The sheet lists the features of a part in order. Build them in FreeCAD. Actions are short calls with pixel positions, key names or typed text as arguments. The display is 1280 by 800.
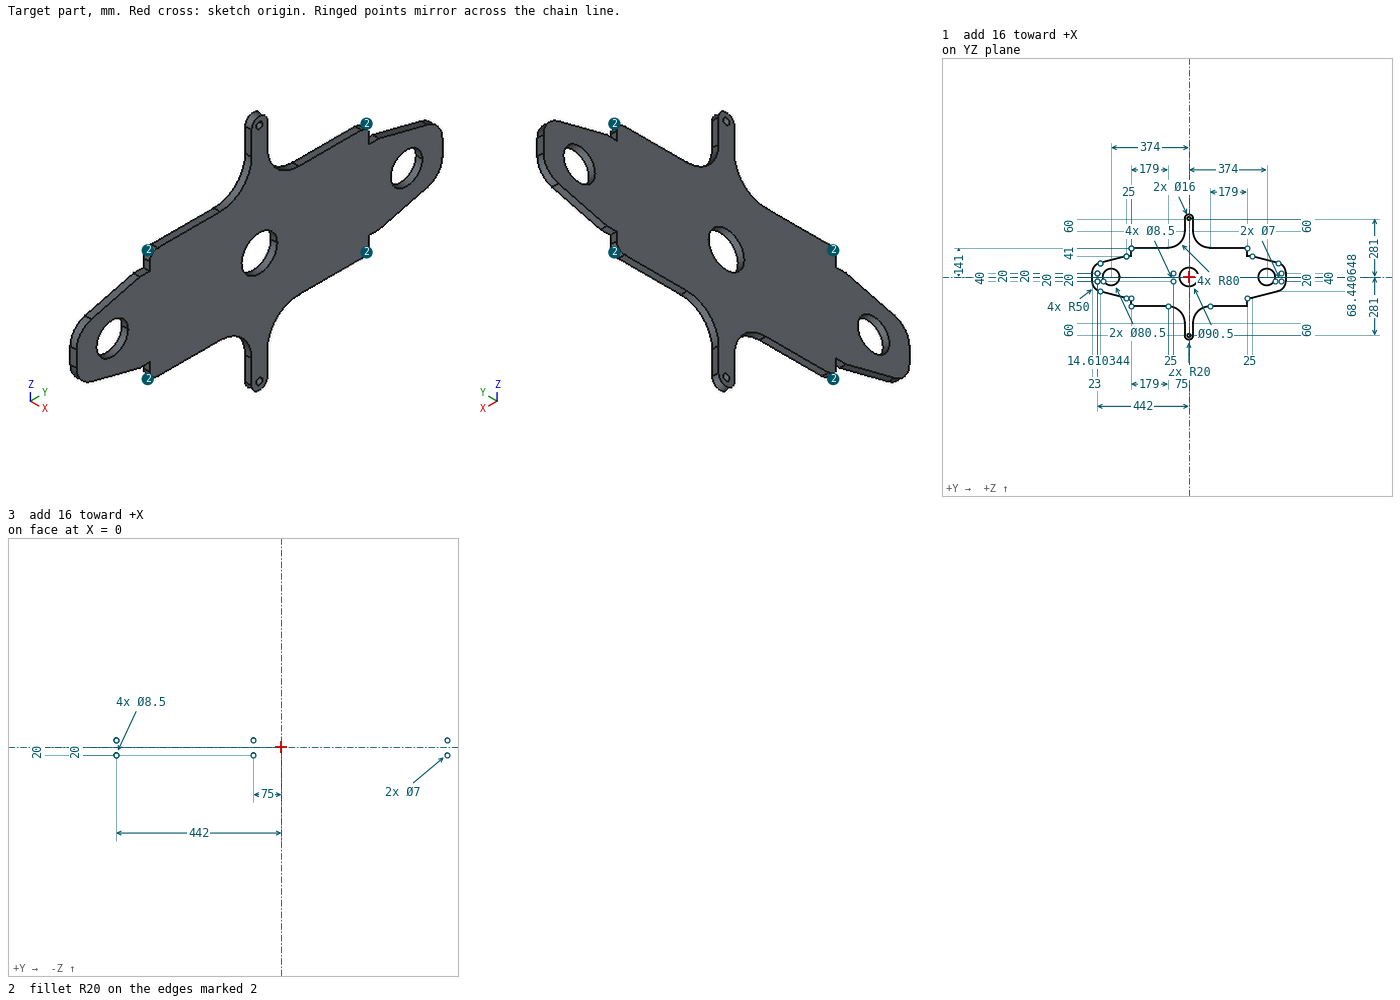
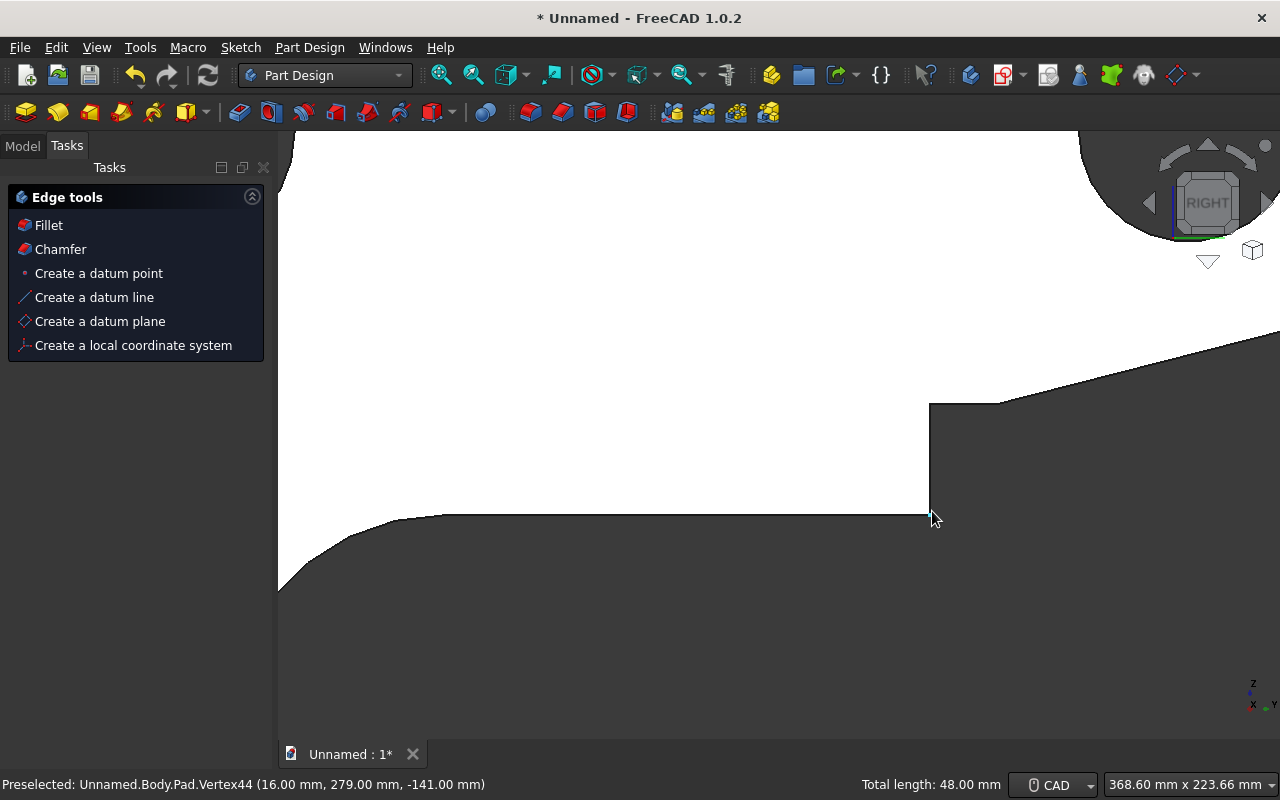
key(v)
key(f)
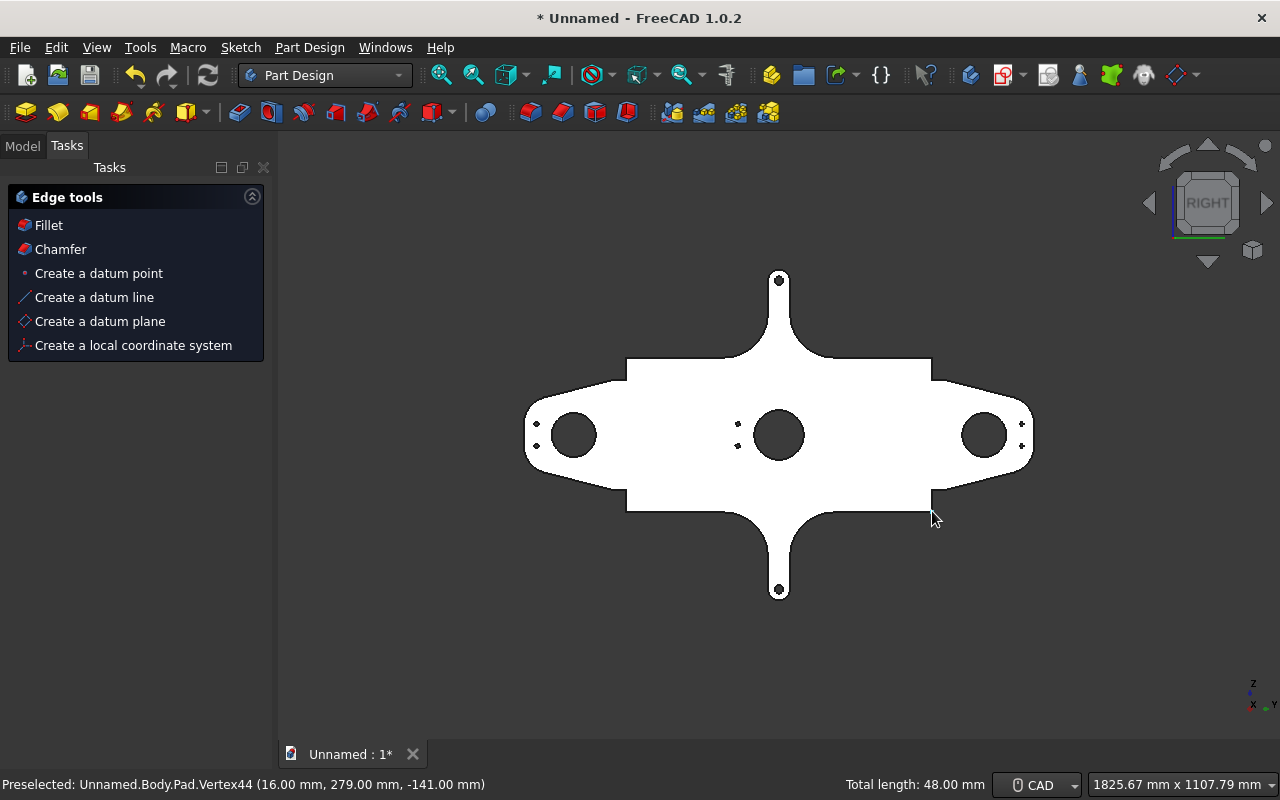
key(5)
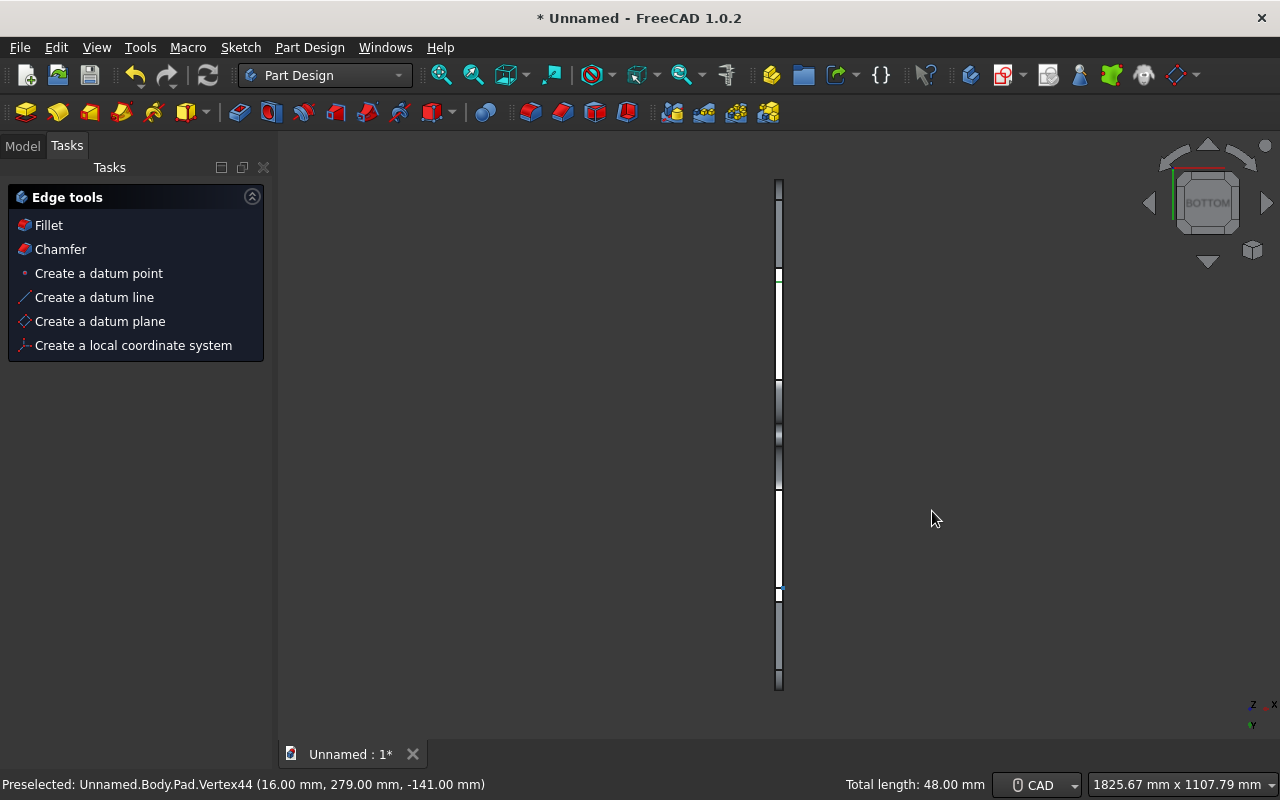
scroll(779, 587, up, 8)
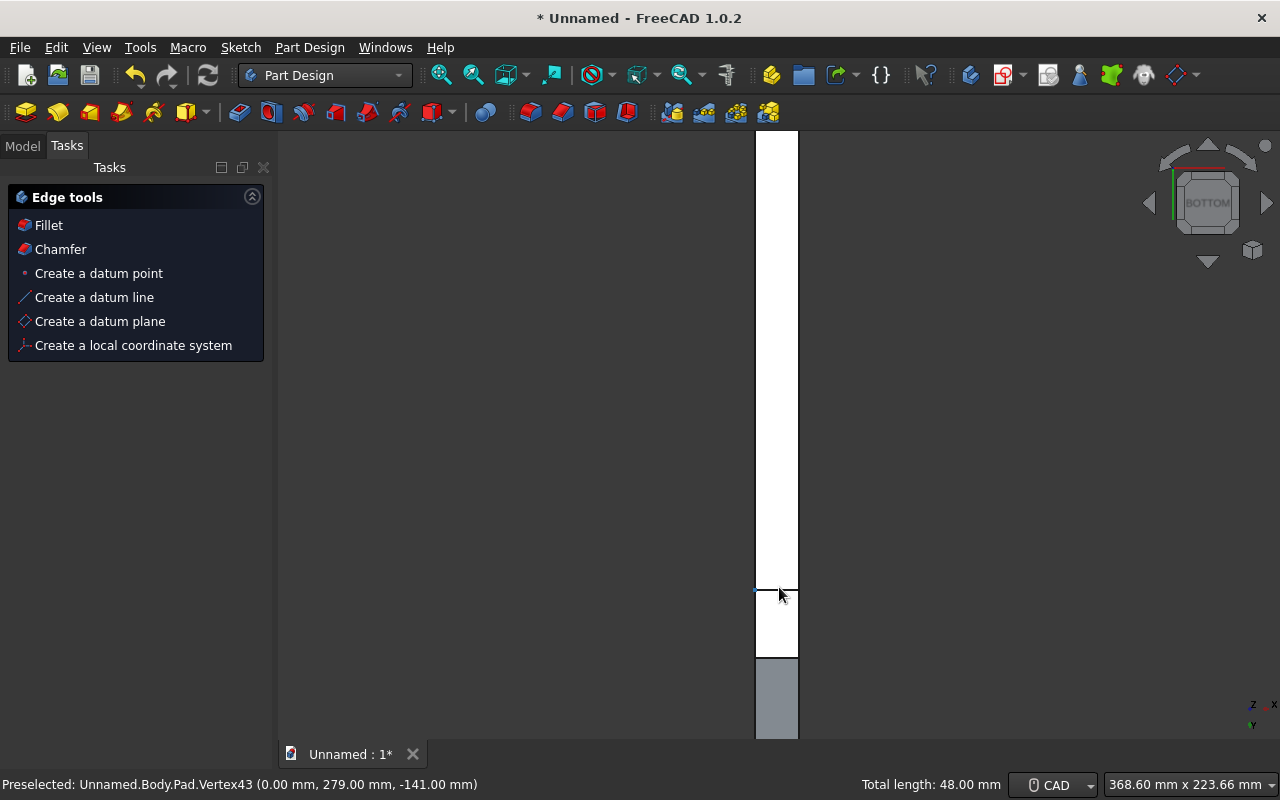
click(777, 589, ctrl)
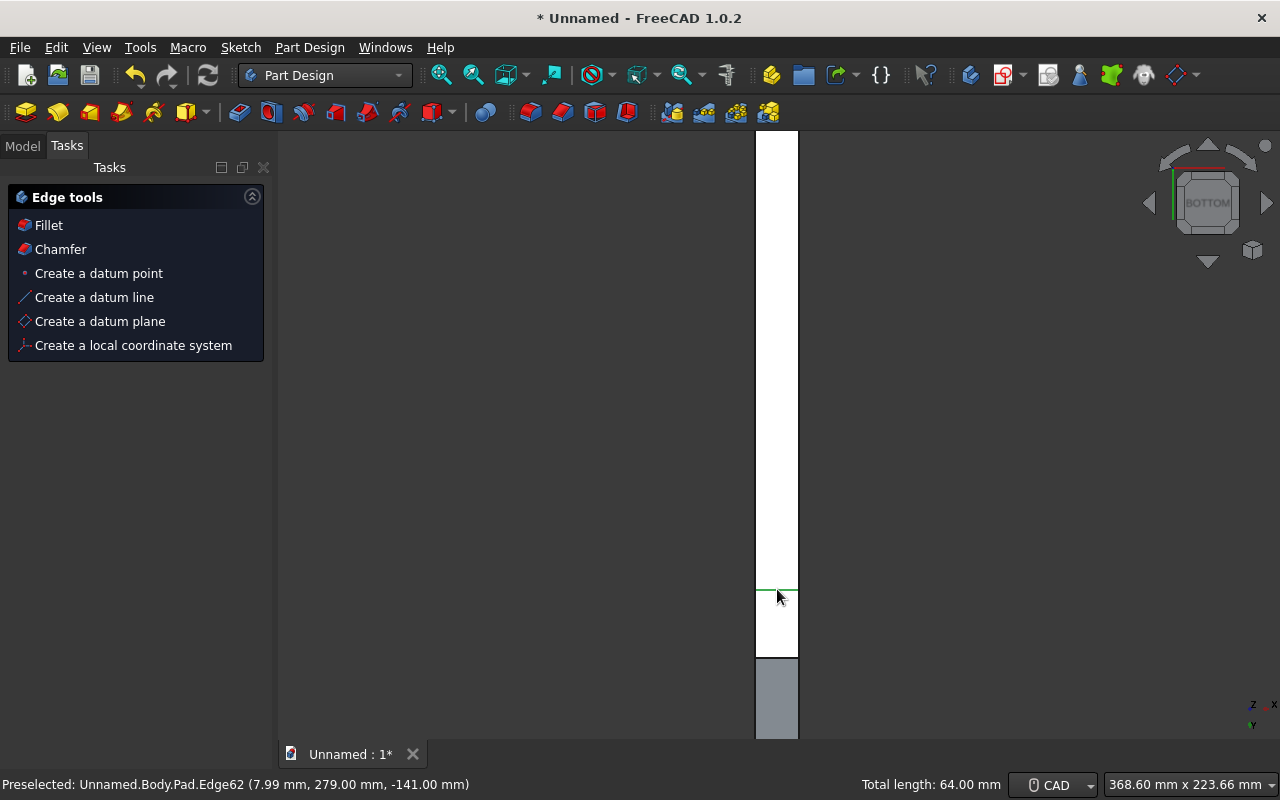
click(532, 112)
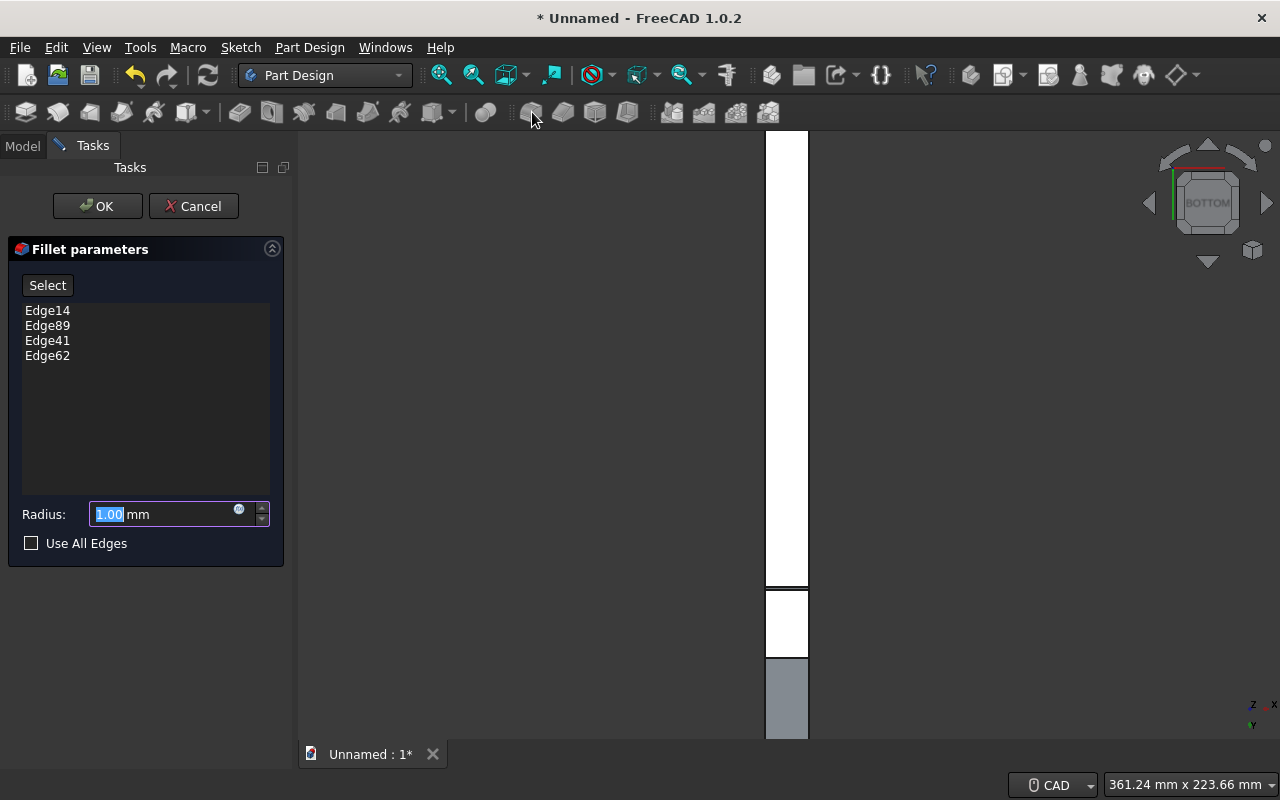
text(20)
key(Tab)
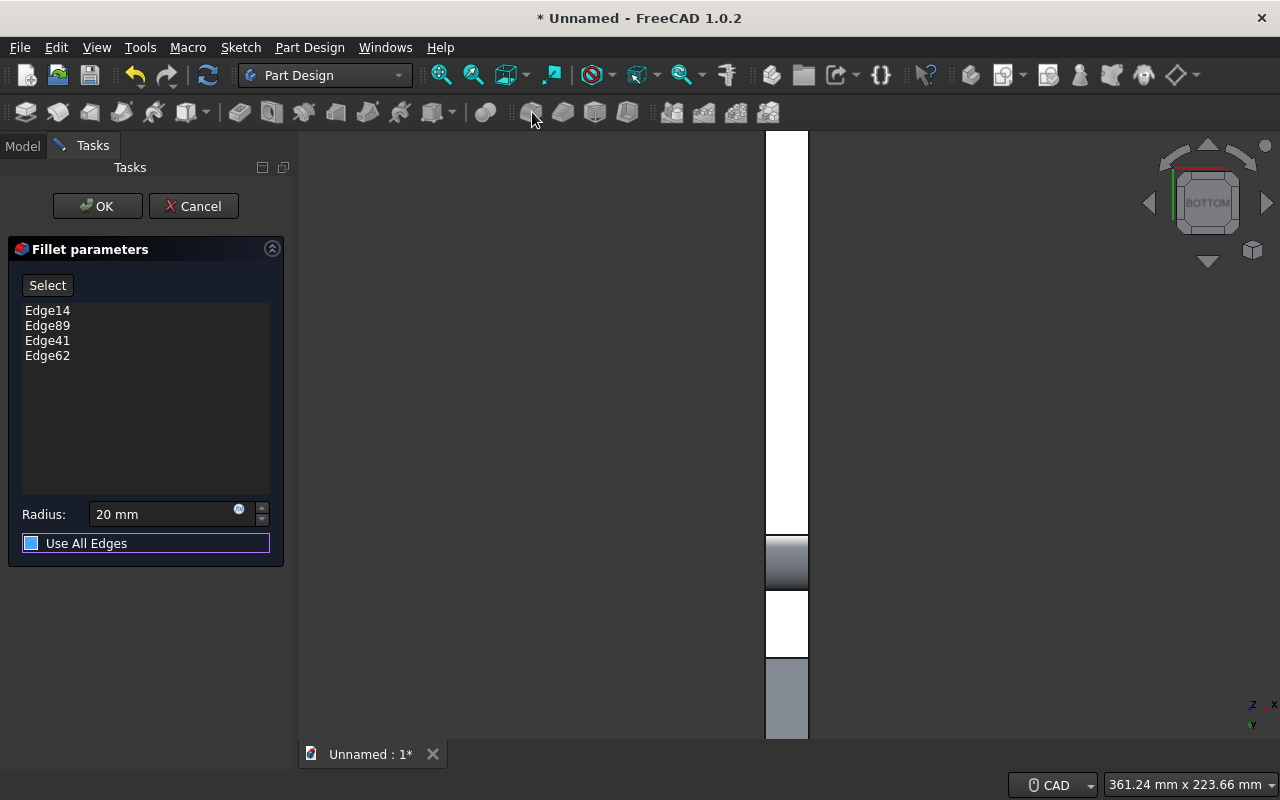
click(98, 206)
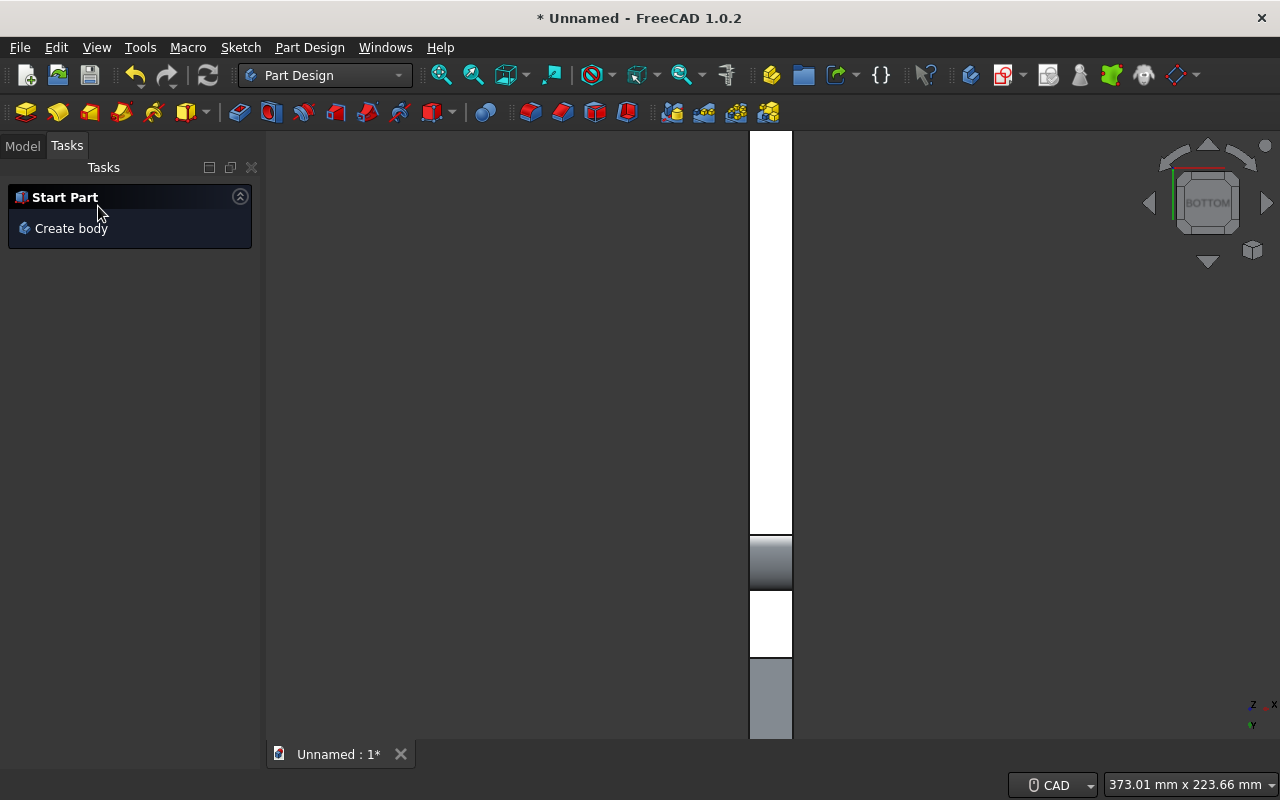
click(442, 76)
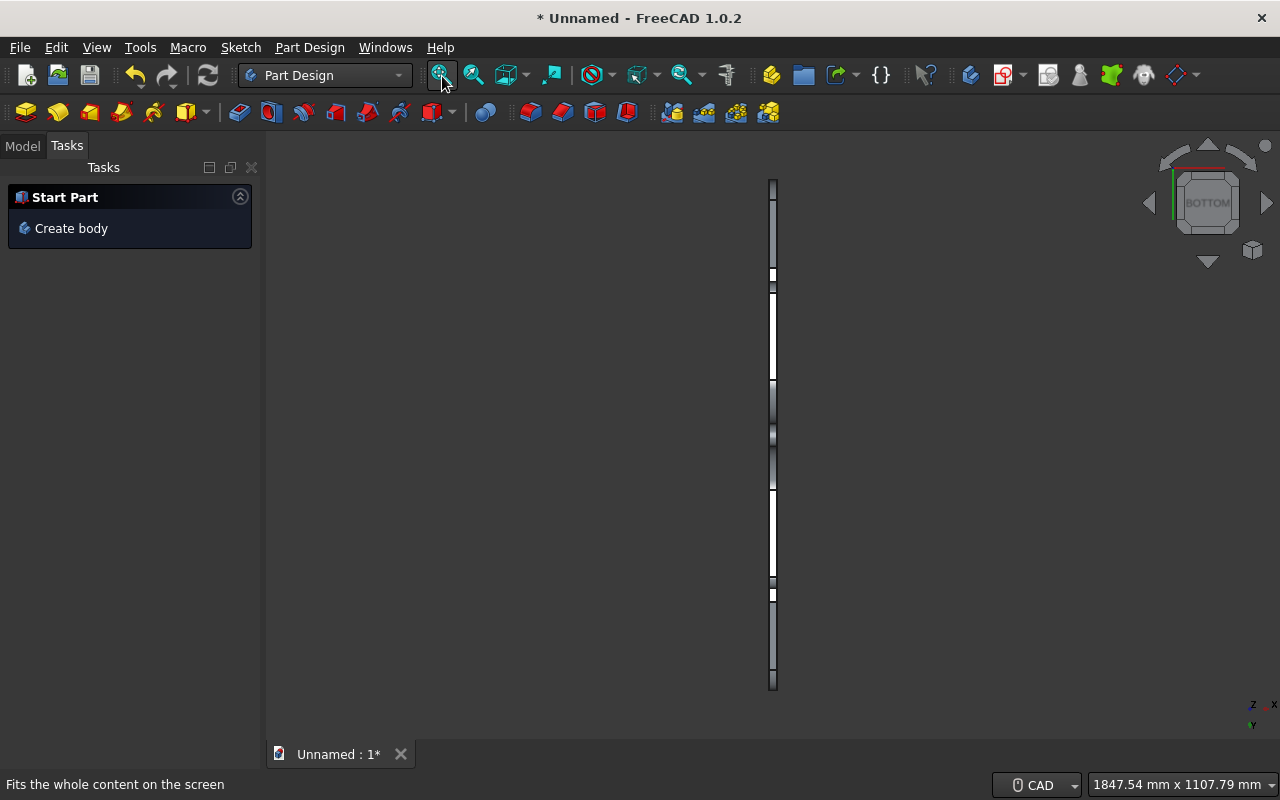
key(6)